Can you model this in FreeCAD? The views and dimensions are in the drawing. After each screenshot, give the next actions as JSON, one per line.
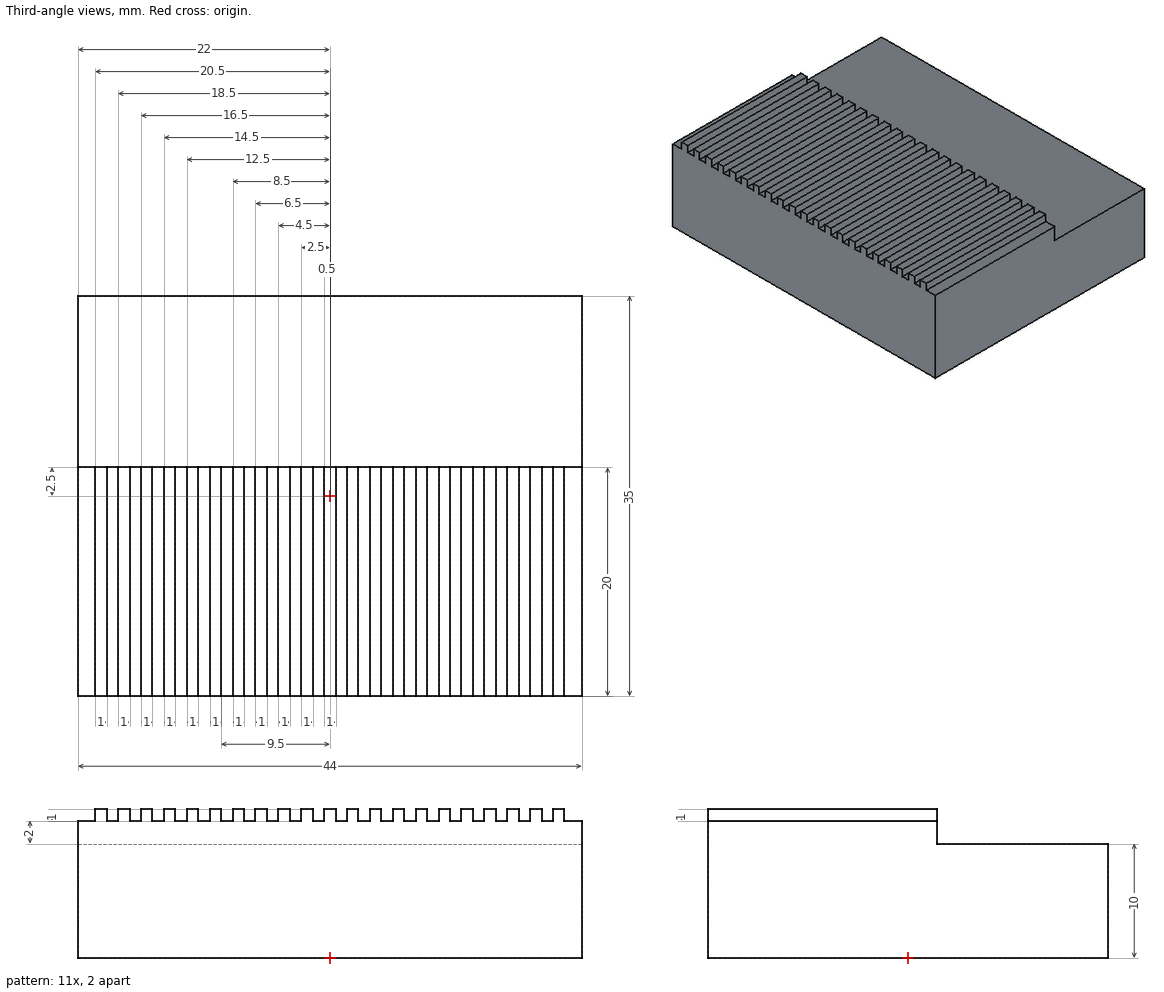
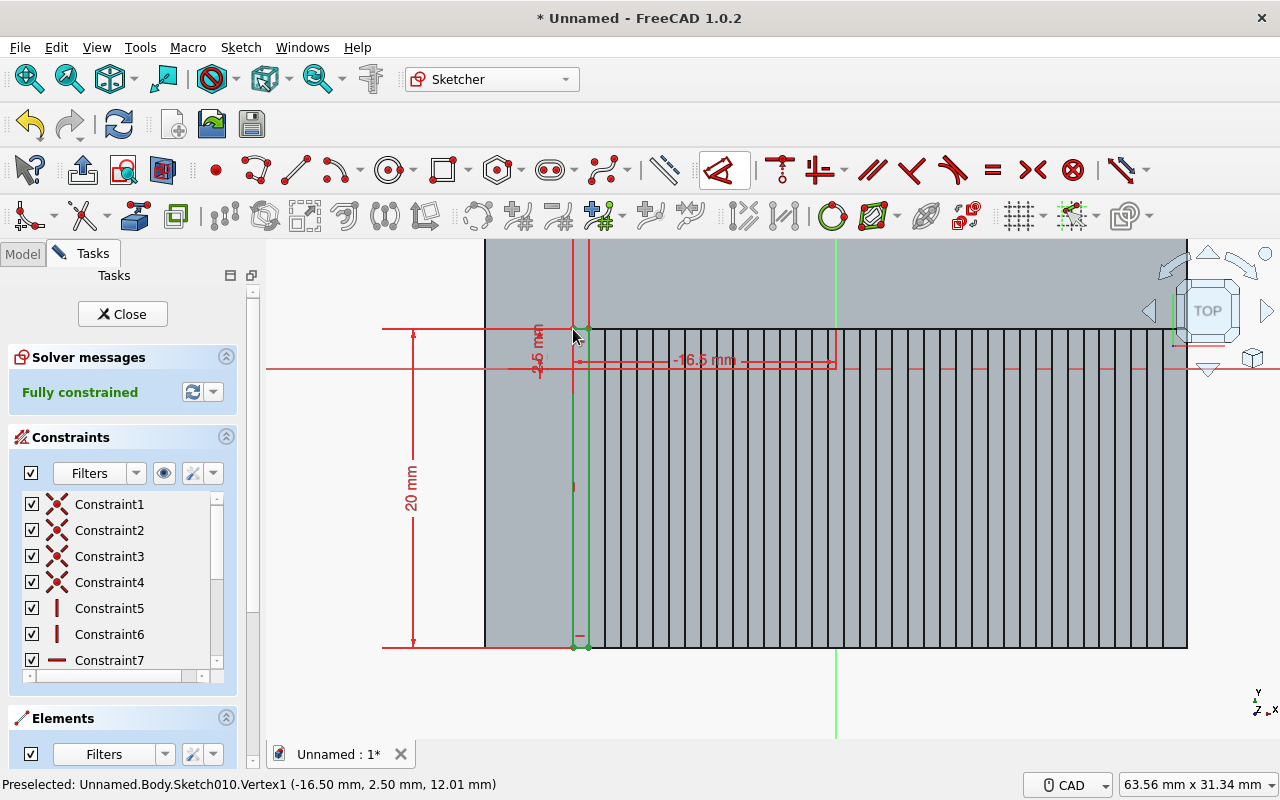
{"action": "left_click", "coordinate": [123, 314]}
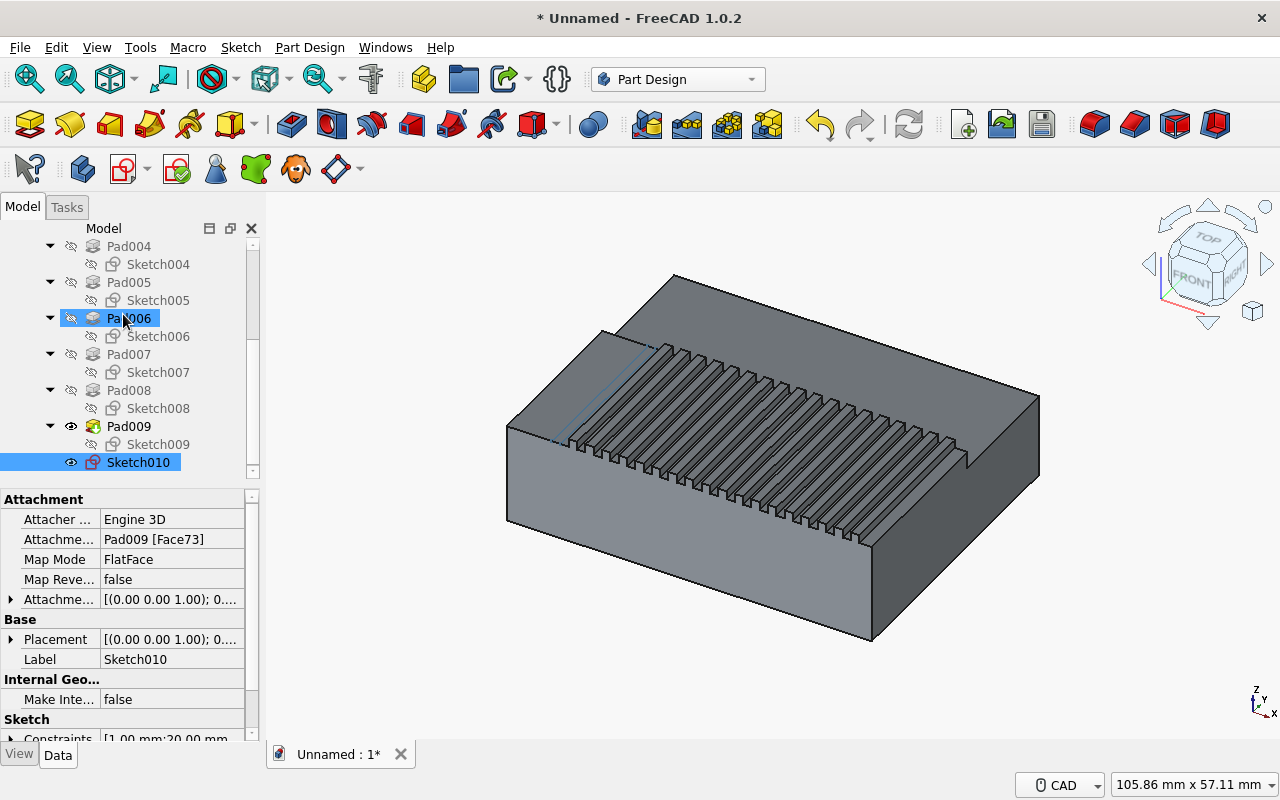
{"action": "left_click", "coordinate": [30, 124]}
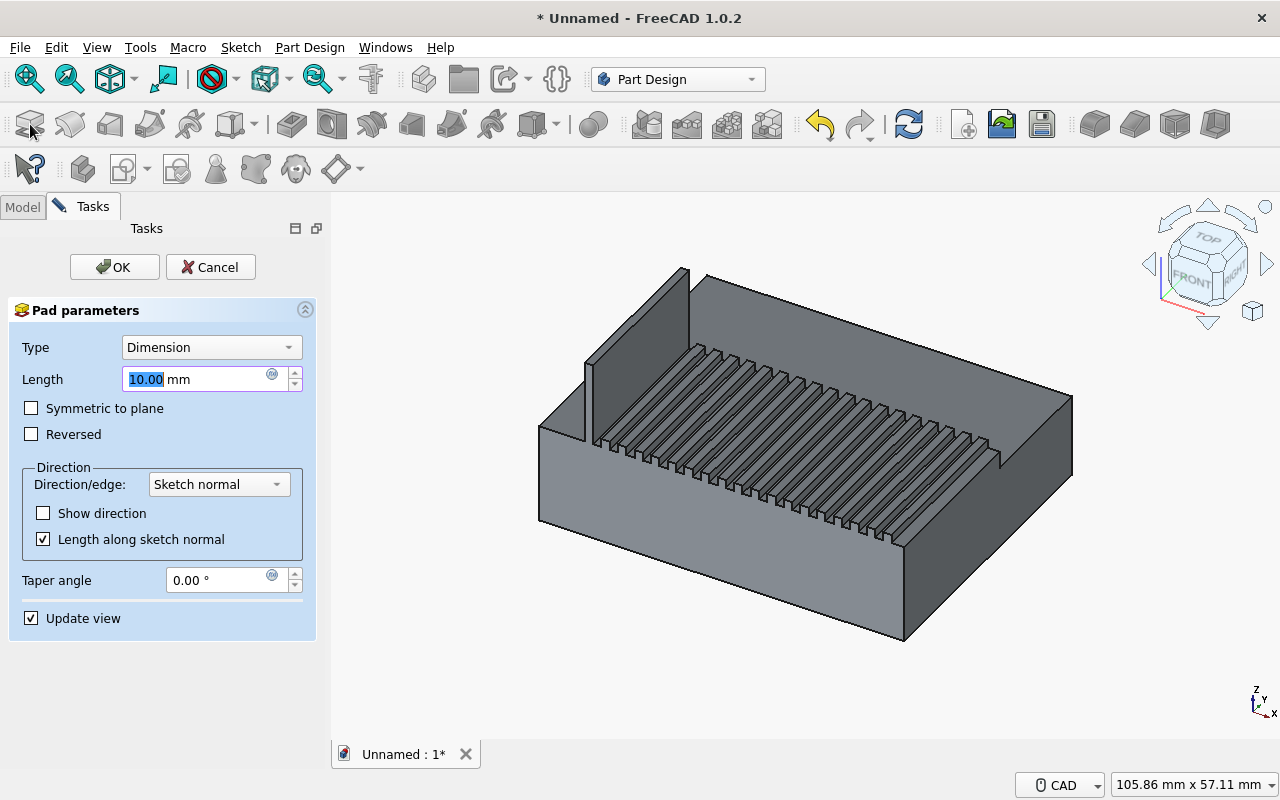
{"action": "type", "text": "1"}
{"action": "key", "text": "Tab"}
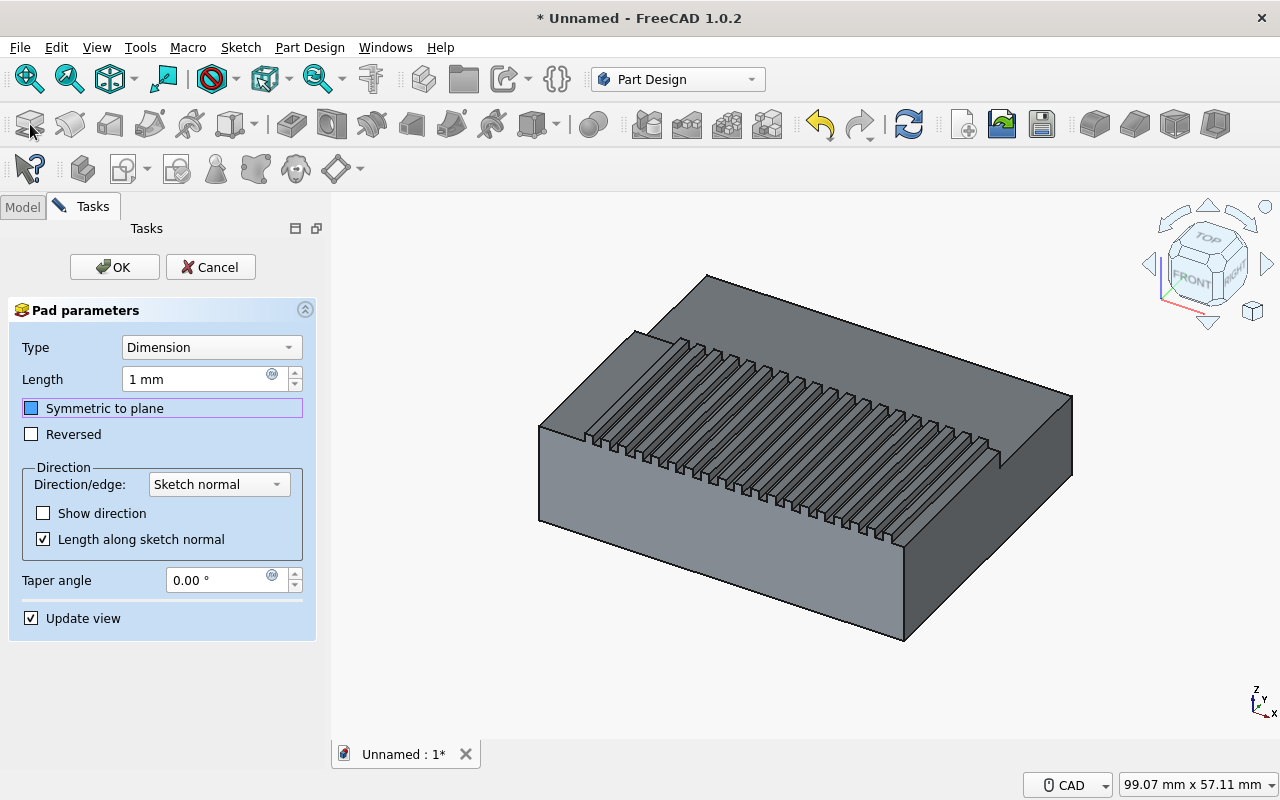
{"action": "left_click", "coordinate": [115, 267]}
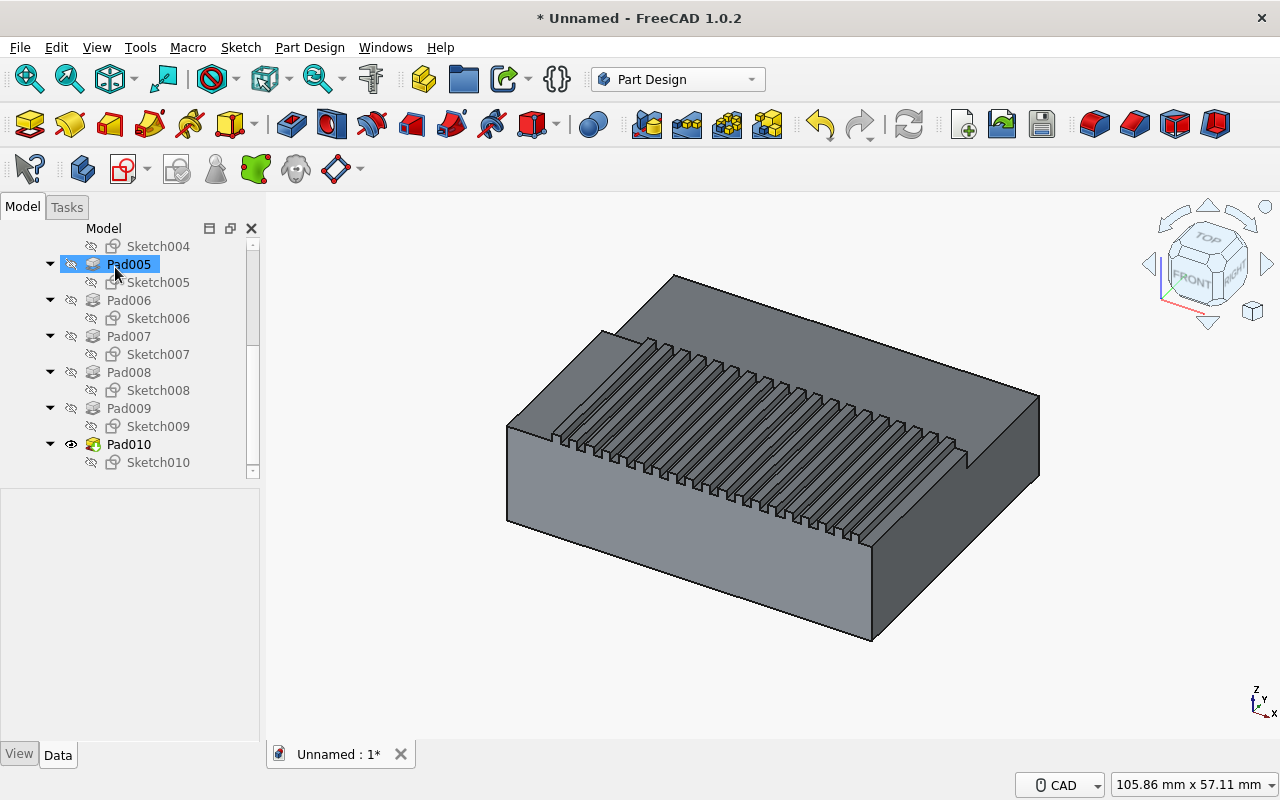
{"action": "left_click", "coordinate": [605, 358]}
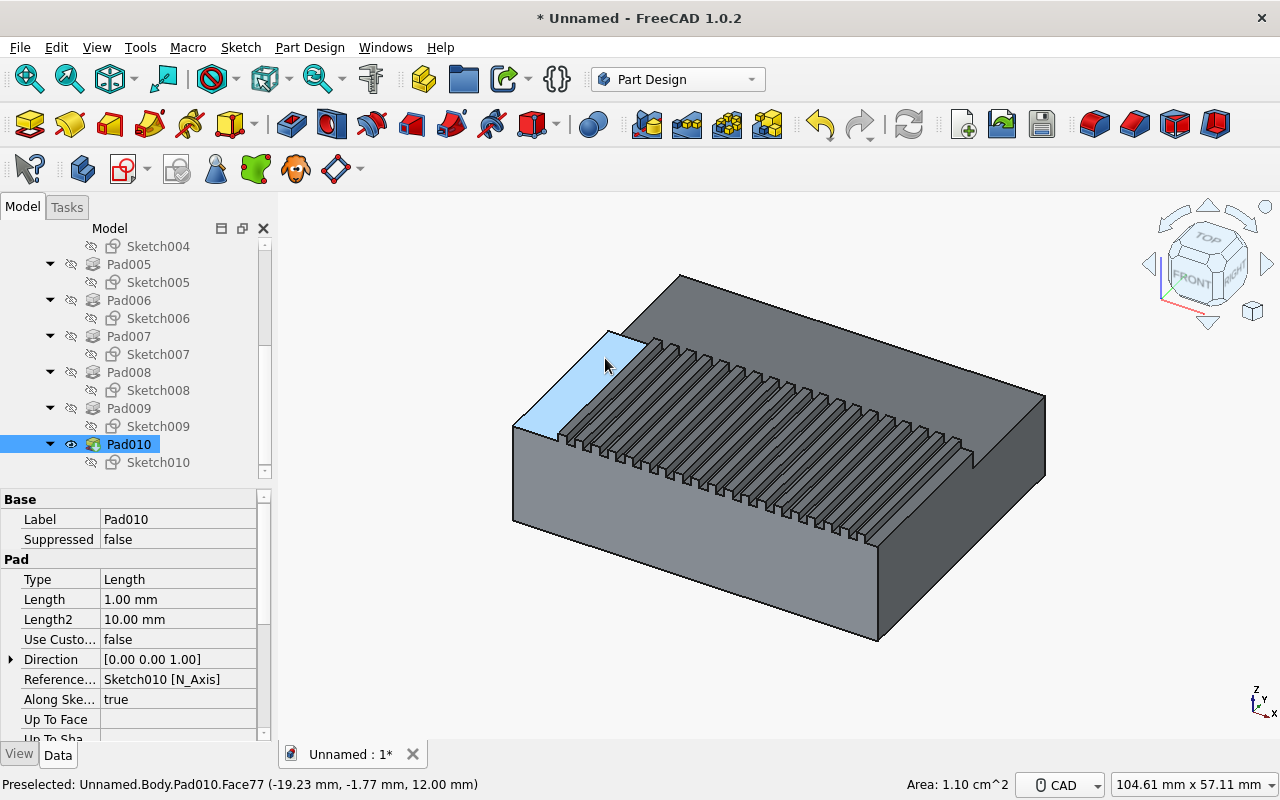
{"action": "left_click", "coordinate": [124, 170]}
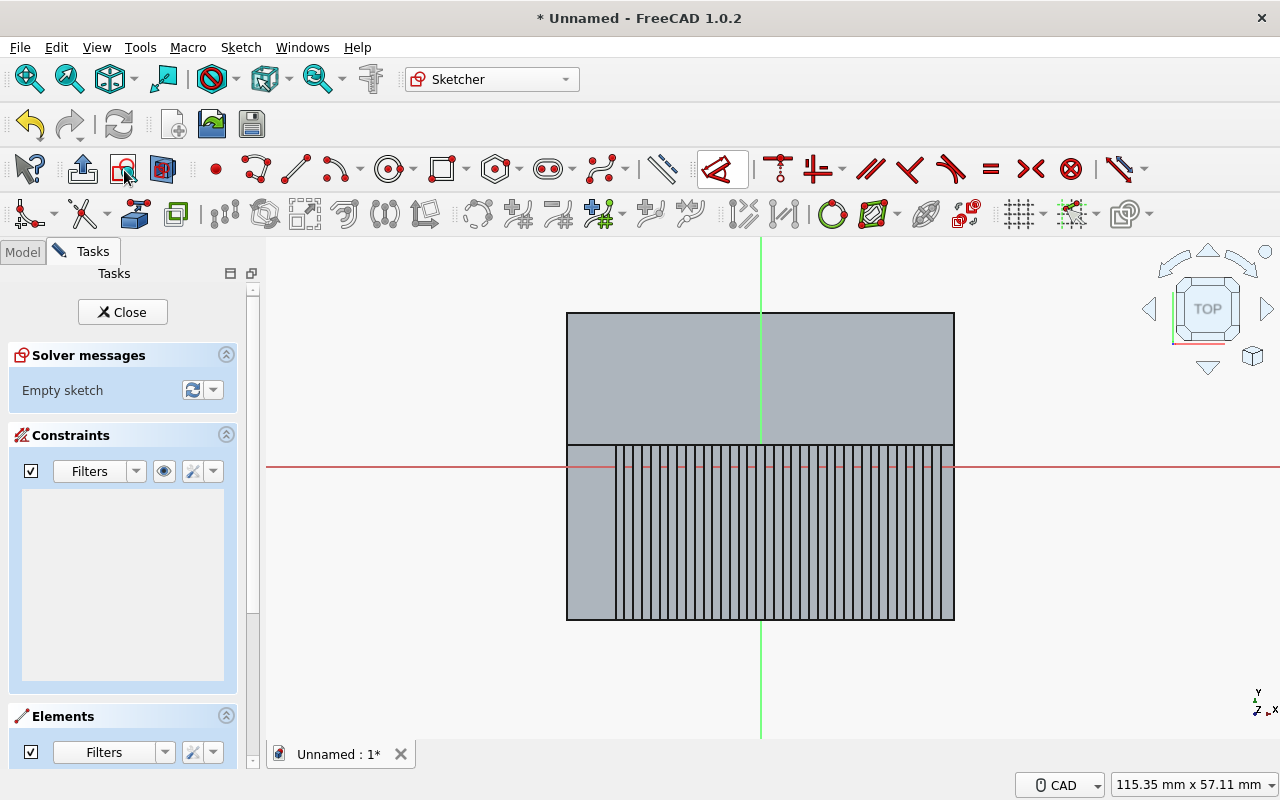
{"action": "scroll", "coordinate": [649, 587], "scroll_direction": "up", "scroll_amount": 3}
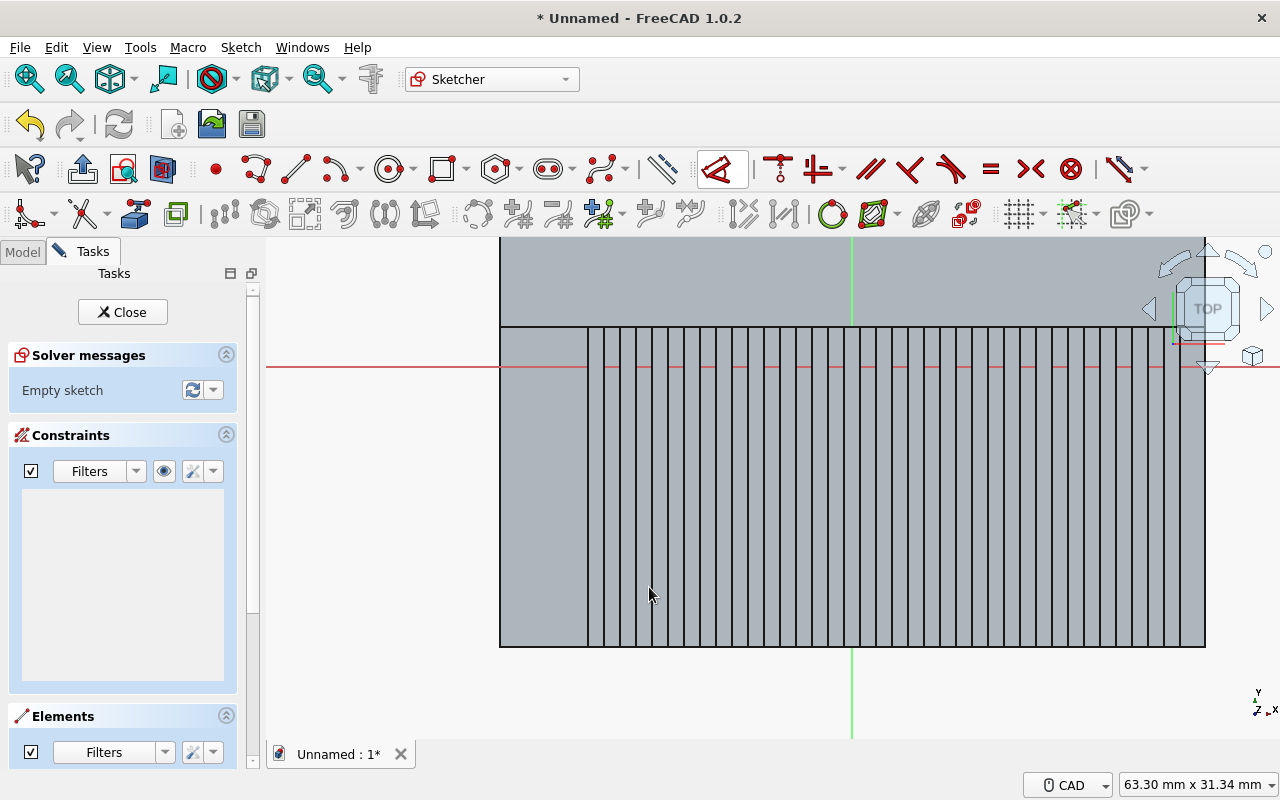
{"action": "left_click", "coordinate": [442, 170]}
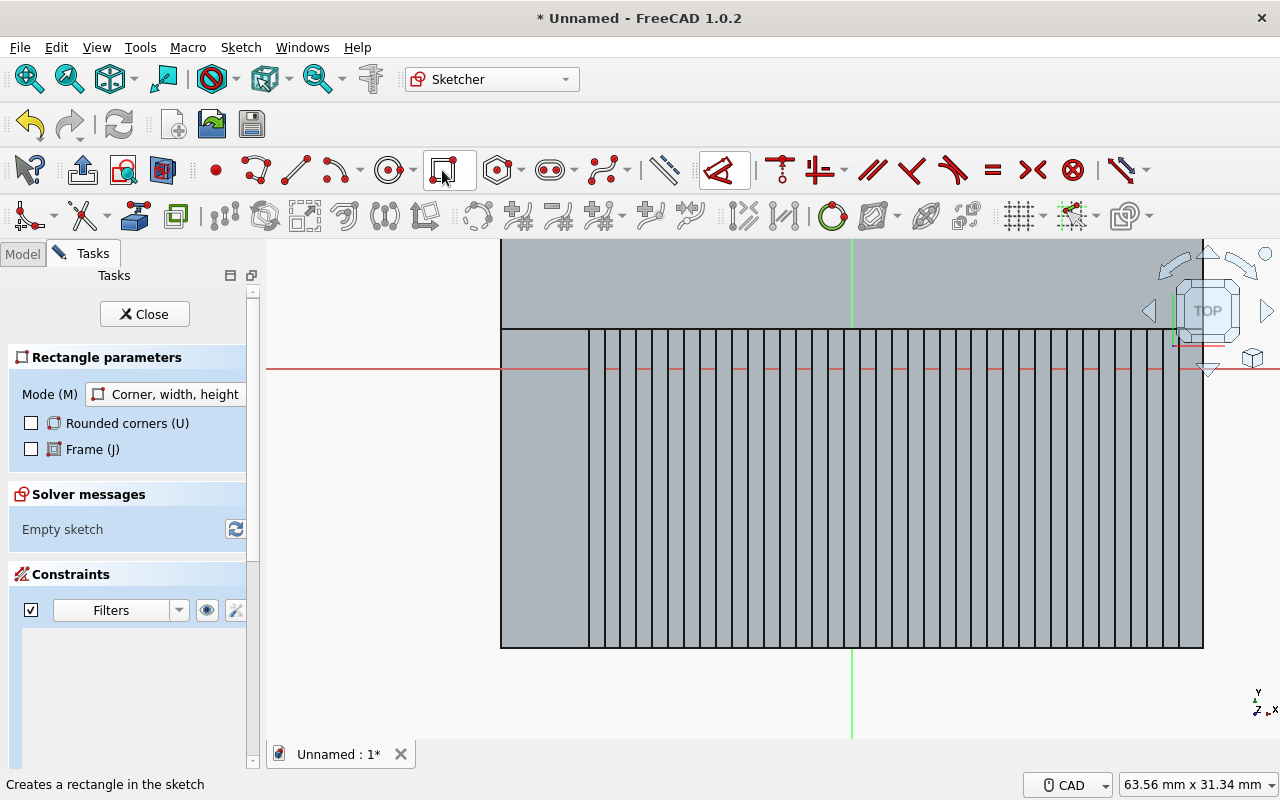
{"action": "left_click", "coordinate": [557, 329]}
{"action": "mouse_move", "coordinate": [573, 648]}